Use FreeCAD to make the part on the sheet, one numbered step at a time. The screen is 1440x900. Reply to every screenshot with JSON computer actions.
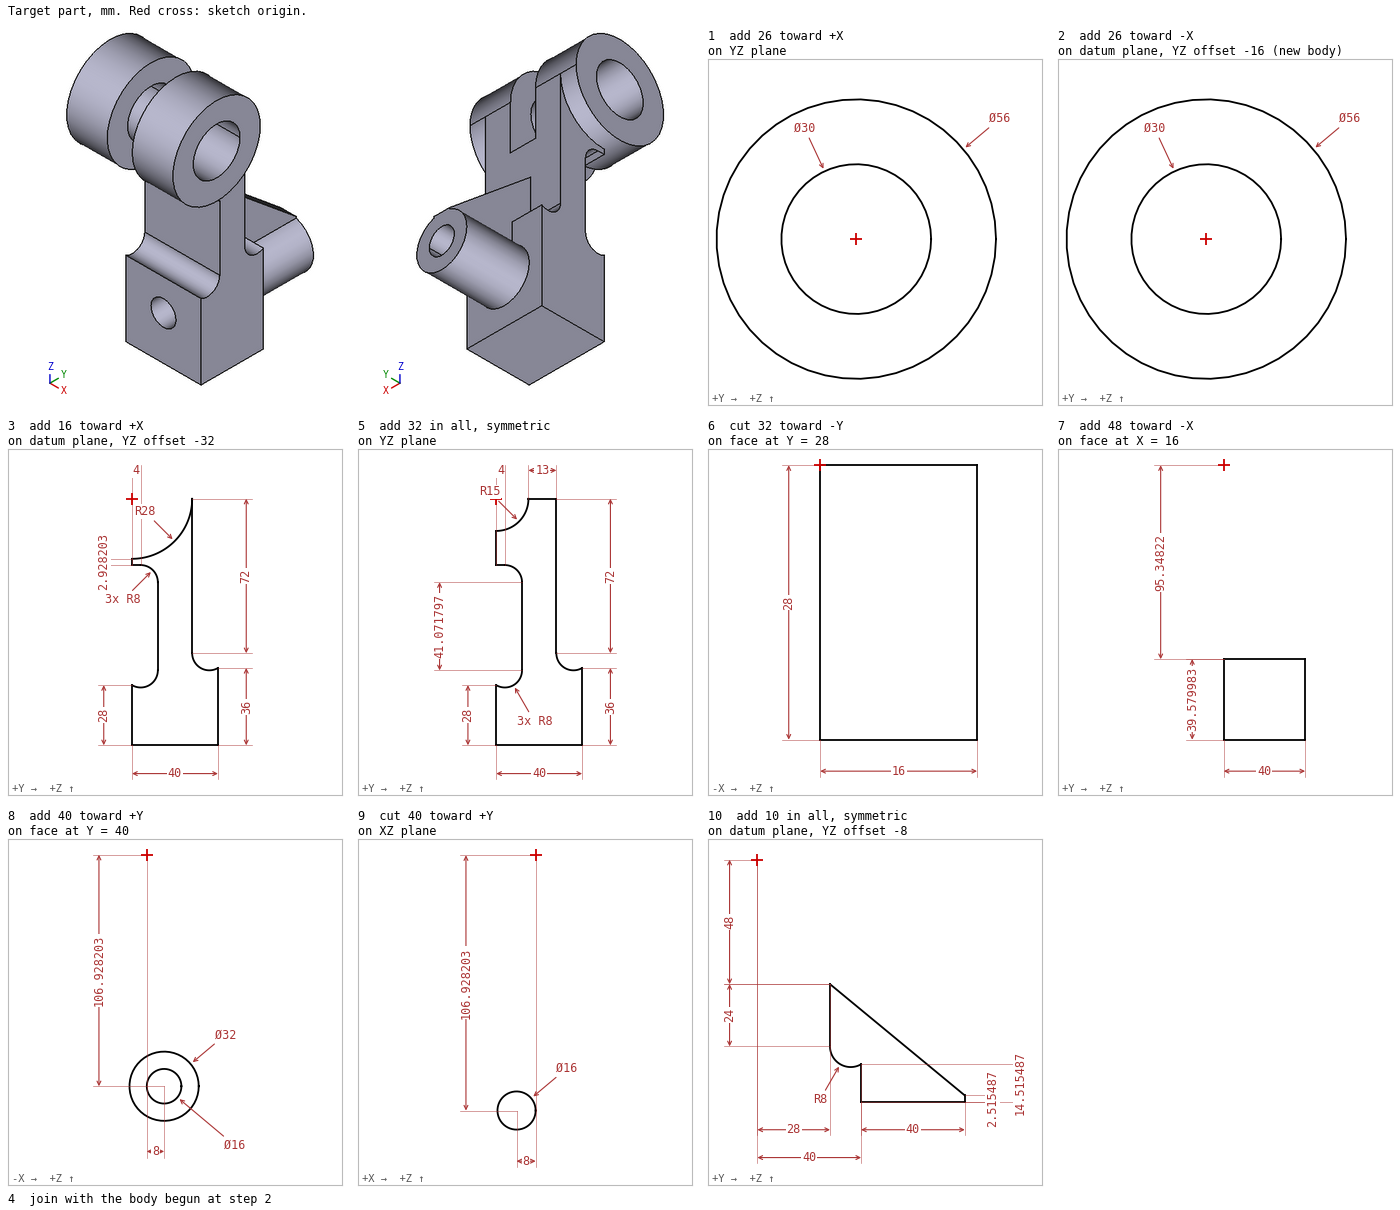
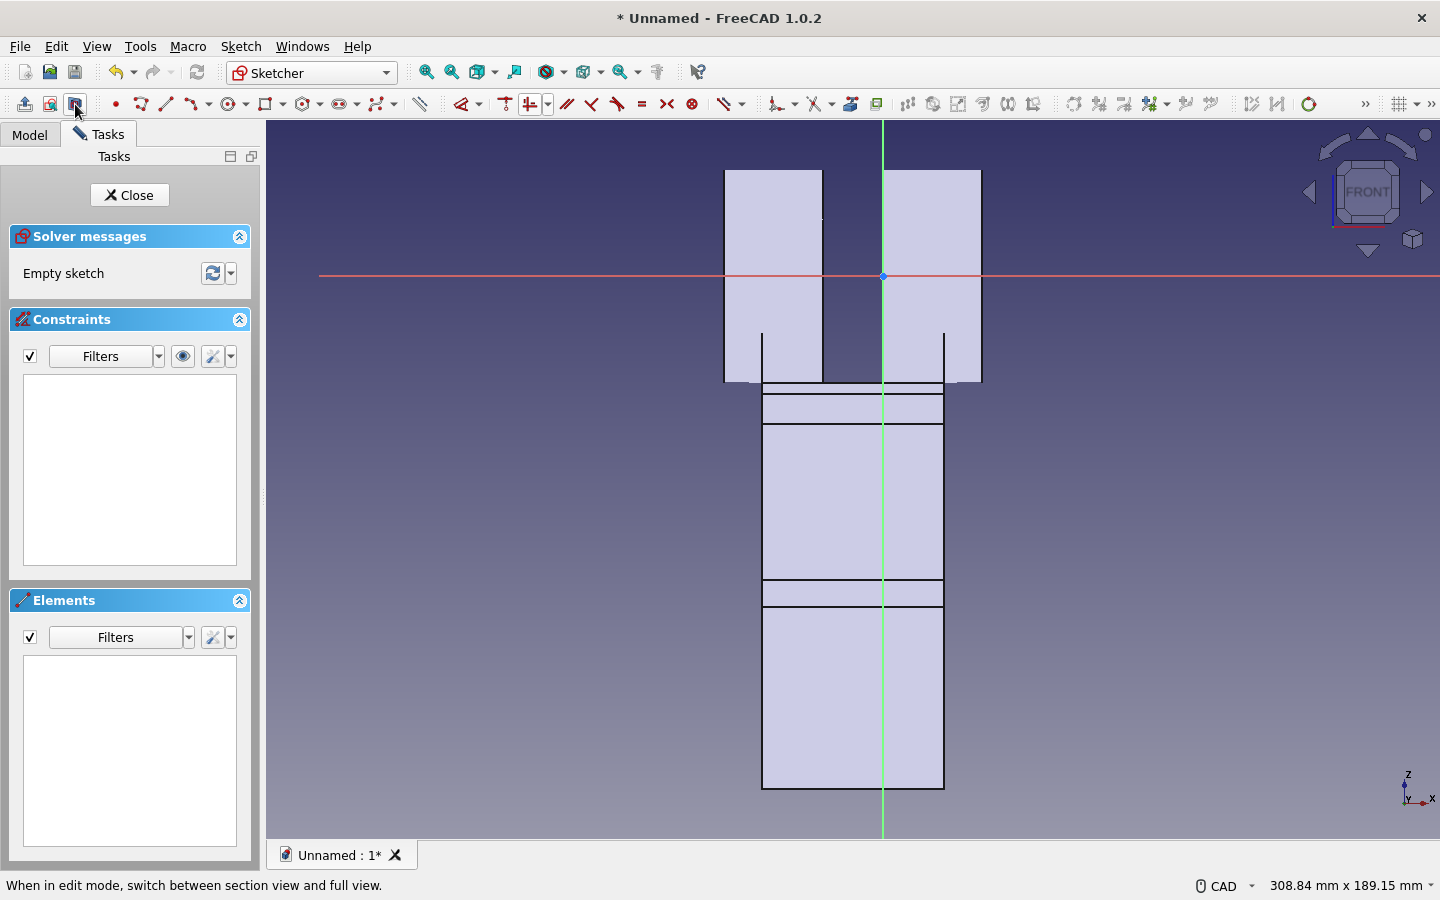
{"action": "scroll", "coordinate": [864, 714], "scroll_direction": "up", "scroll_amount": 10}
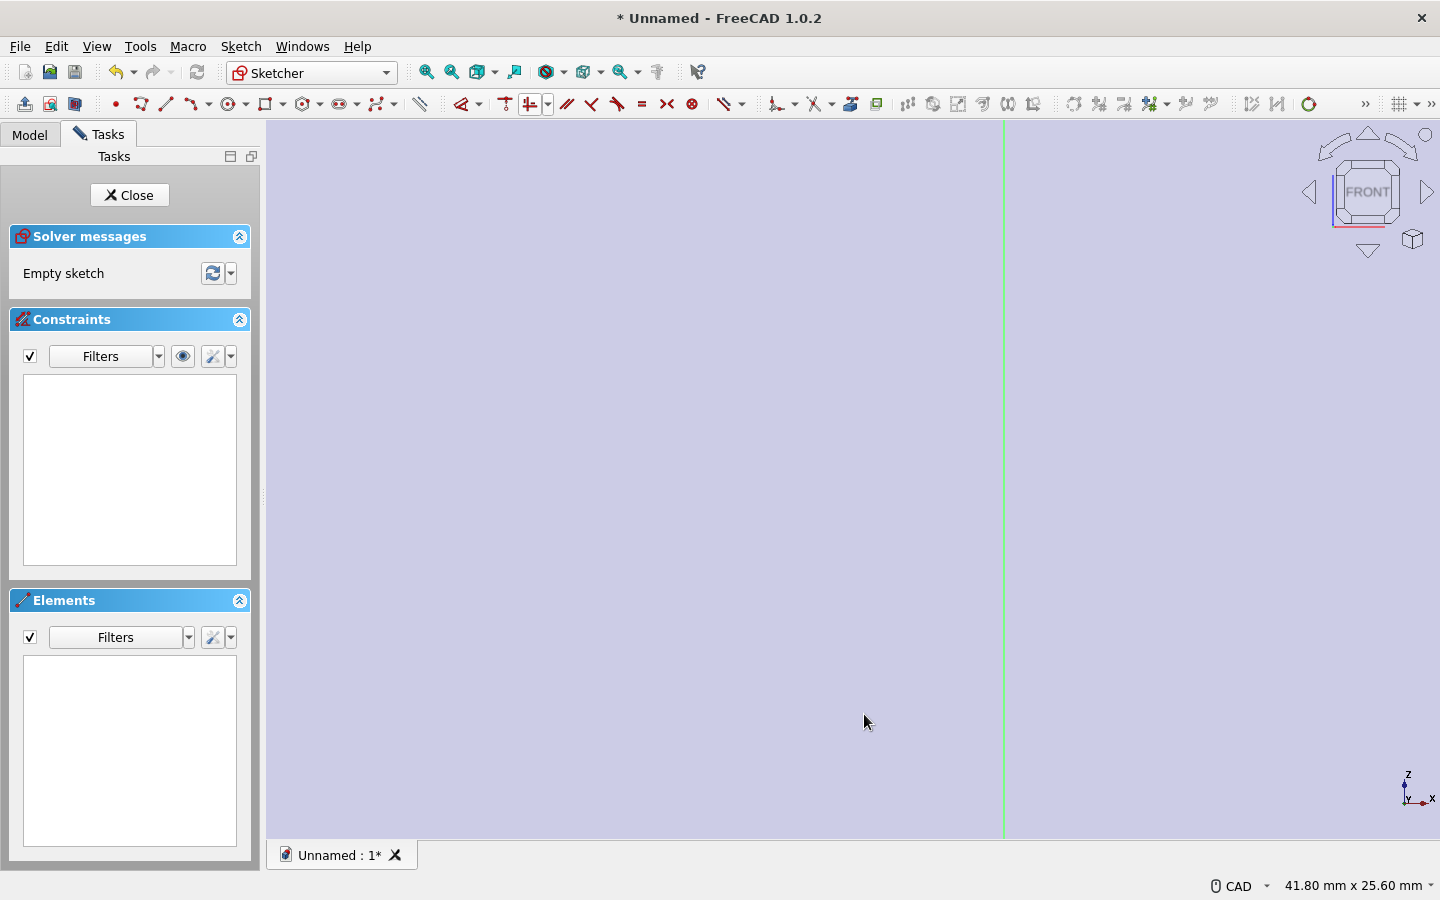
{"action": "key", "text": "g c"}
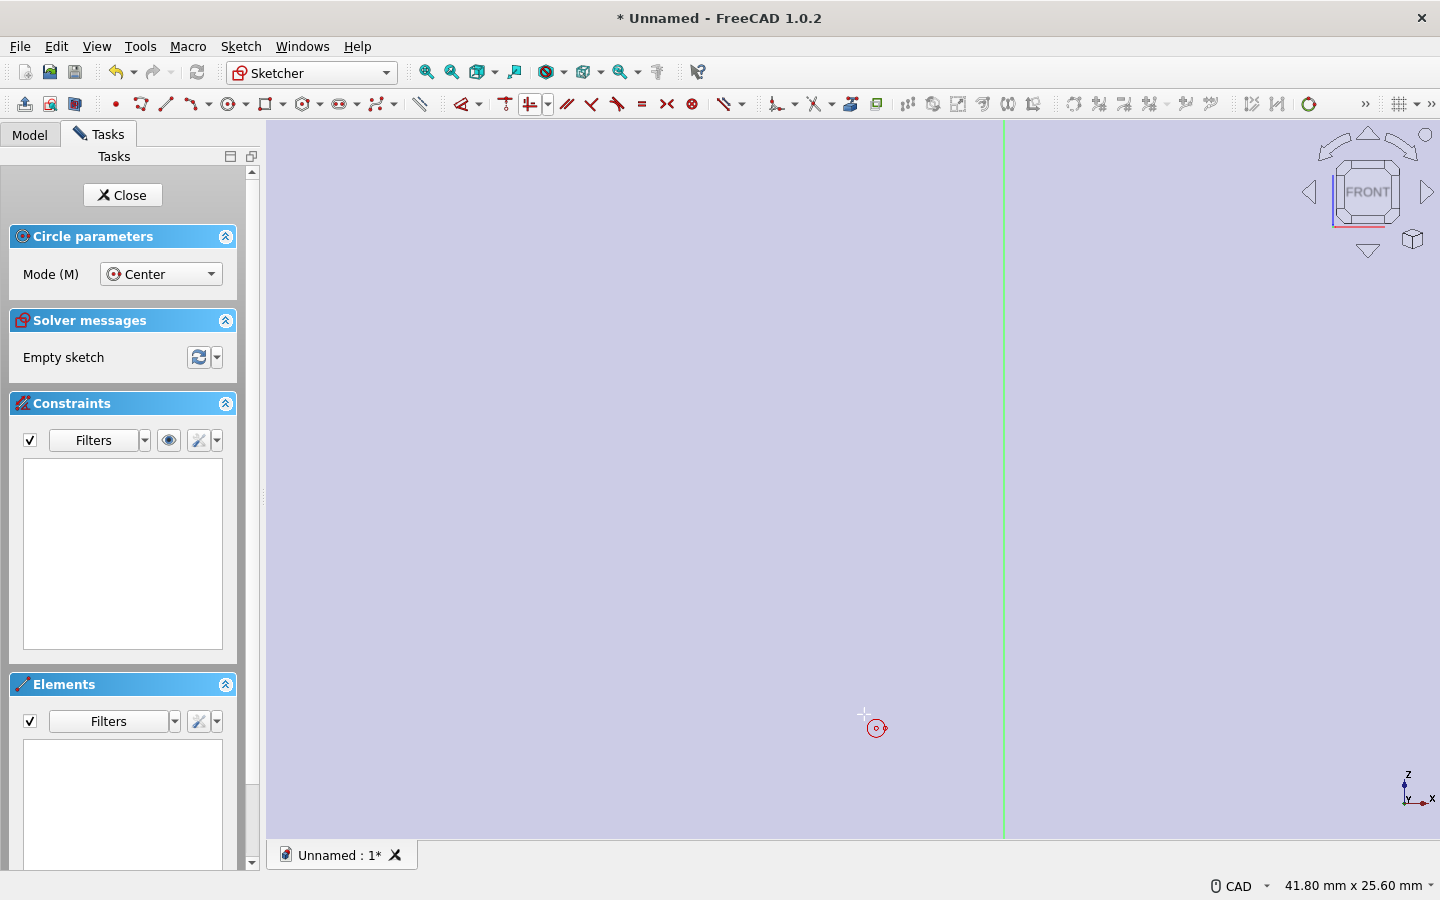
{"action": "left_click", "coordinate": [779, 477]}
{"action": "left_click", "coordinate": [938, 318]}
{"action": "key", "text": "Escape"}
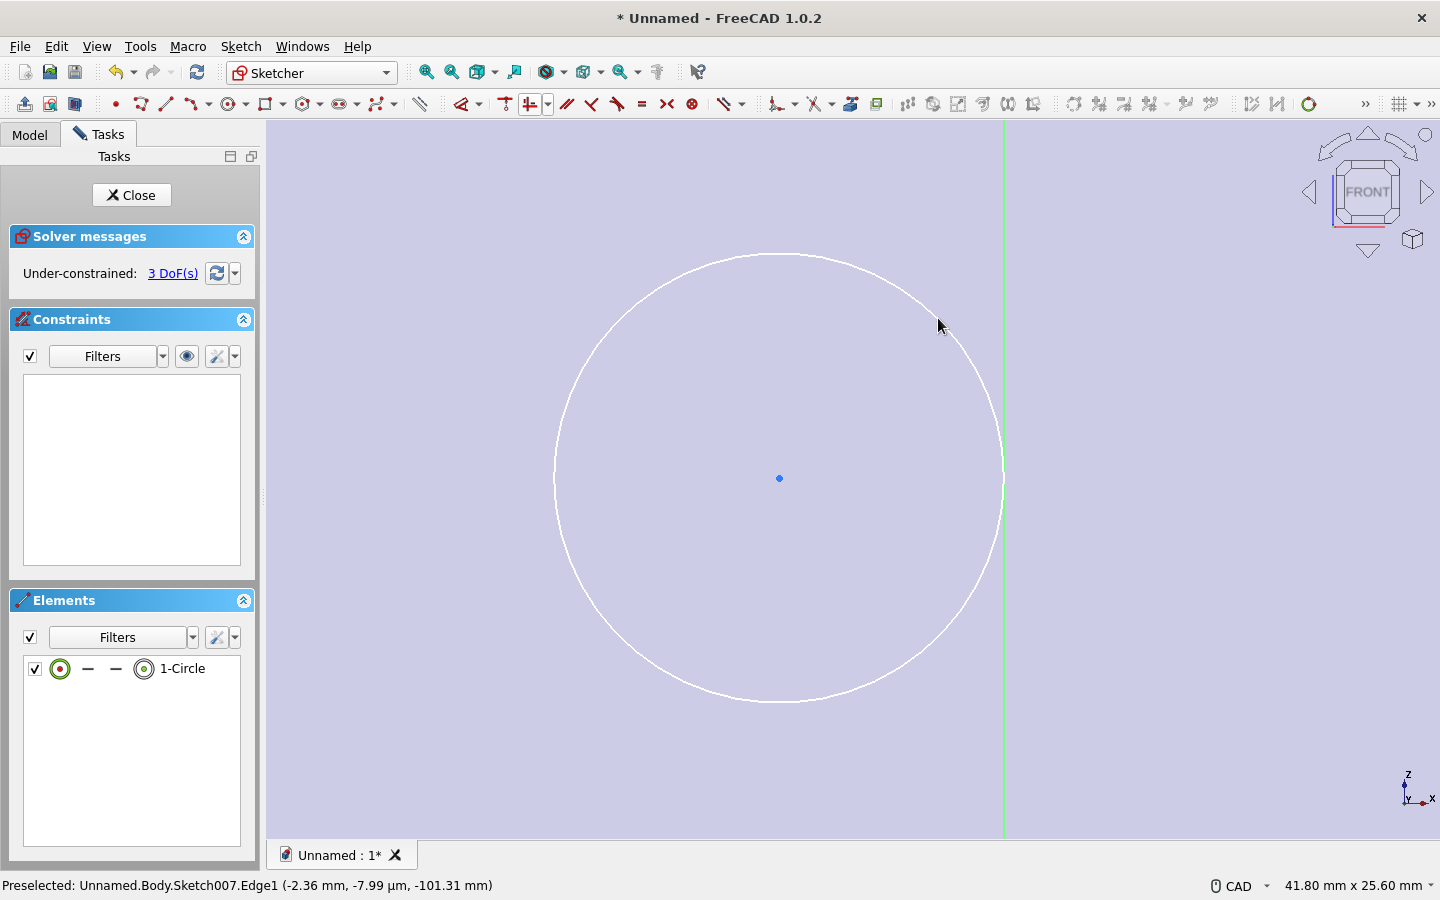
{"action": "key", "text": "d"}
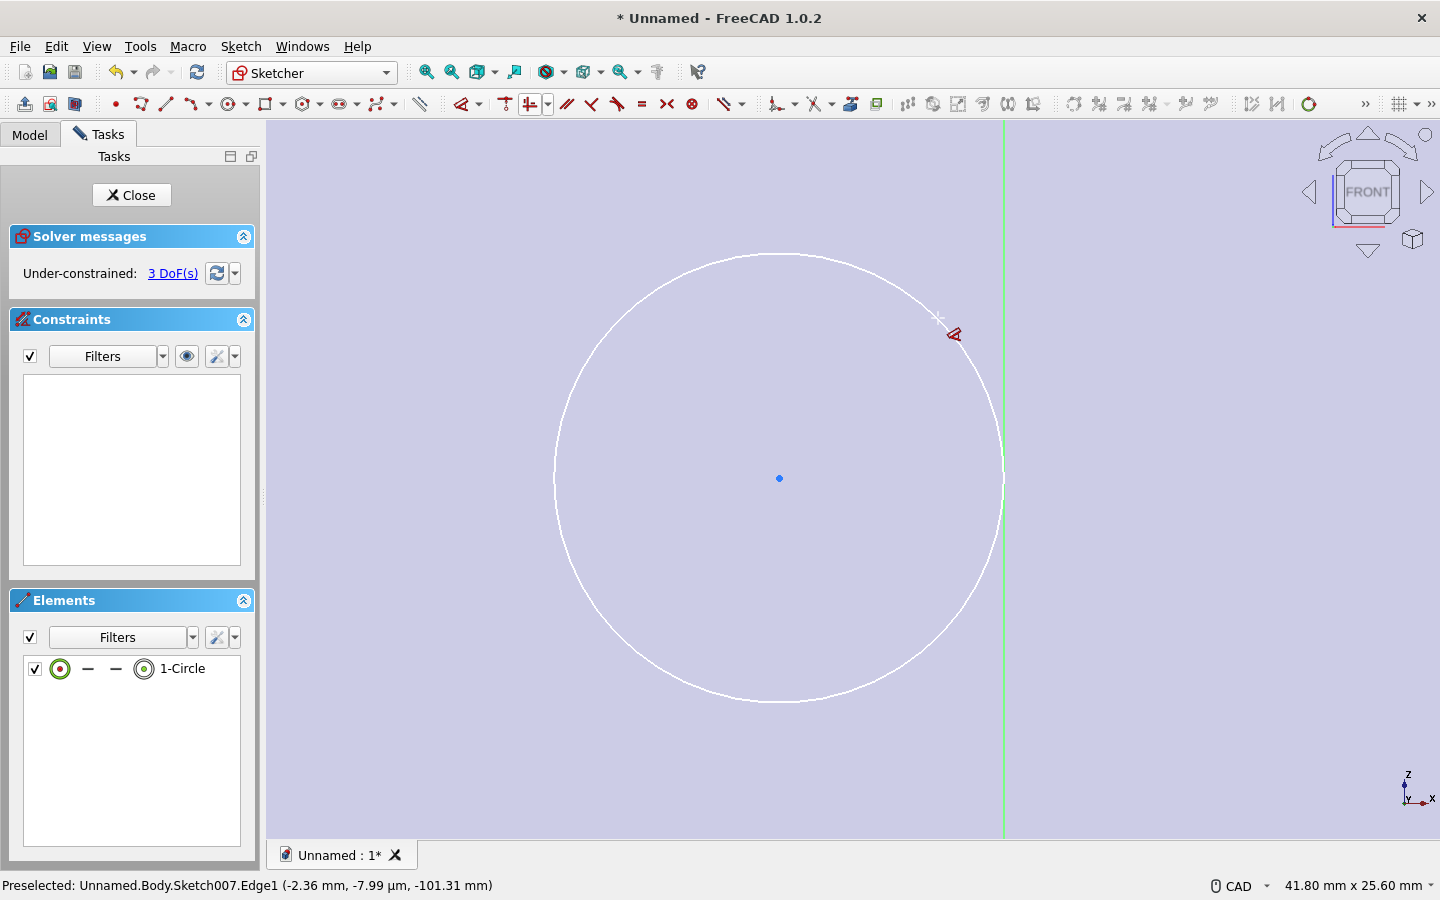
{"action": "left_click", "coordinate": [938, 319]}
{"action": "left_click", "coordinate": [961, 296]}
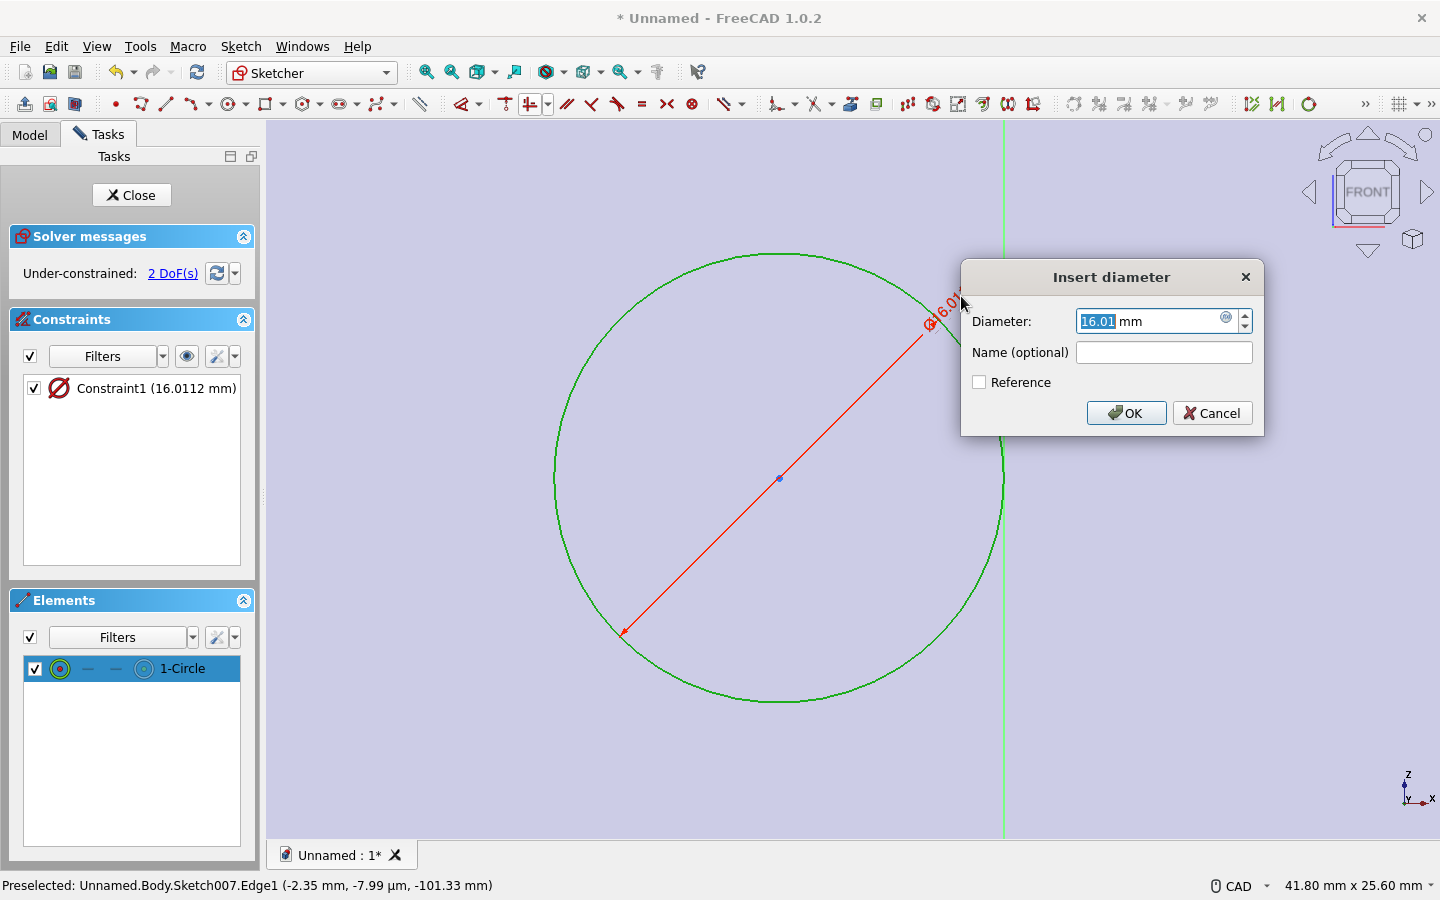
{"action": "type", "text": "16"}
{"action": "key", "text": "Return"}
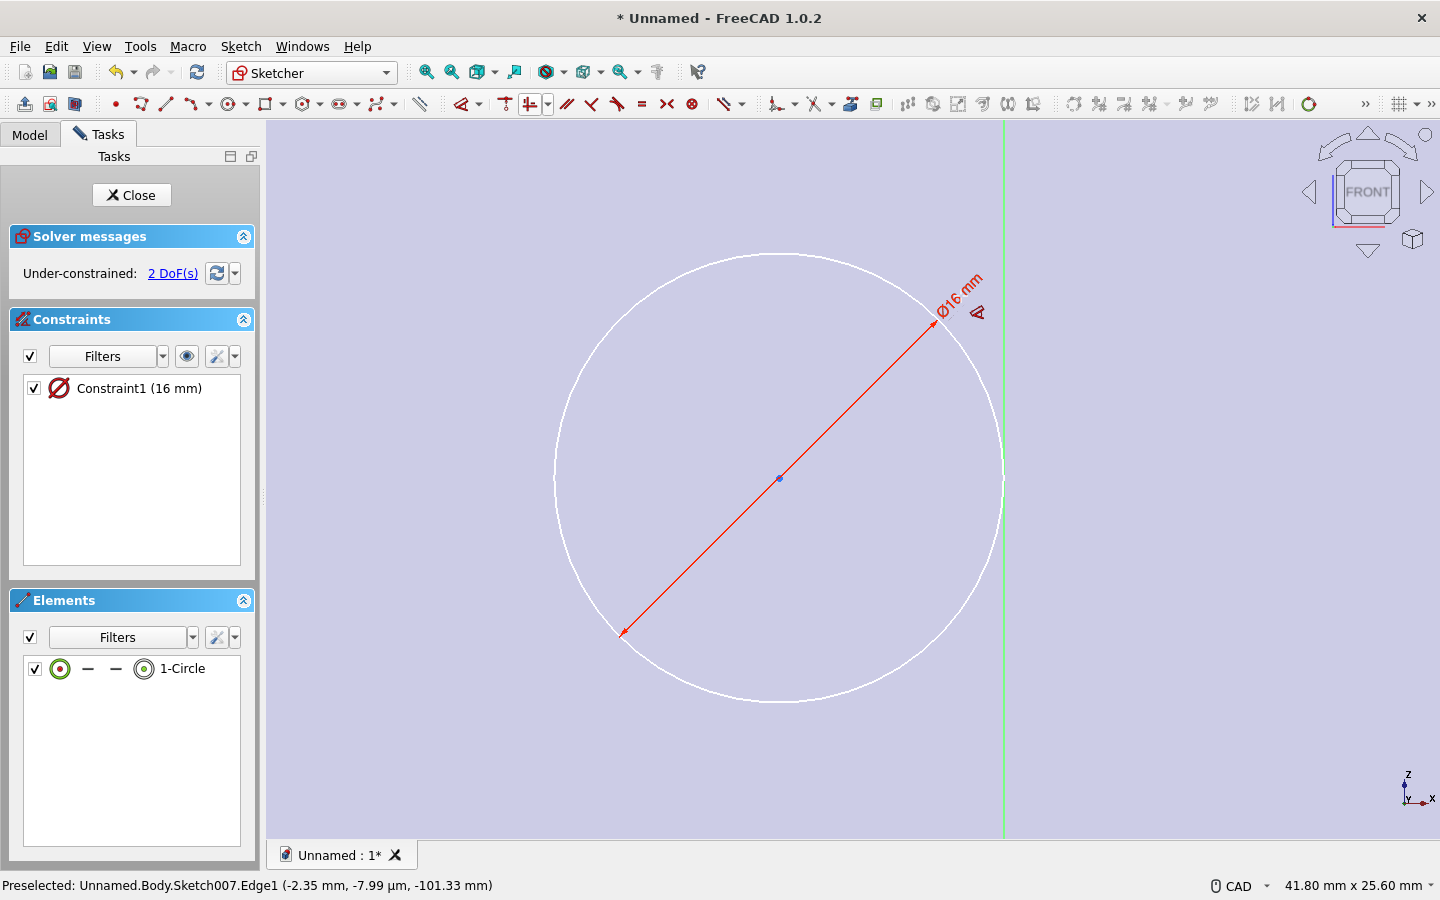
{"action": "left_click", "coordinate": [779, 478]}
{"action": "left_click", "coordinate": [892, 512]}